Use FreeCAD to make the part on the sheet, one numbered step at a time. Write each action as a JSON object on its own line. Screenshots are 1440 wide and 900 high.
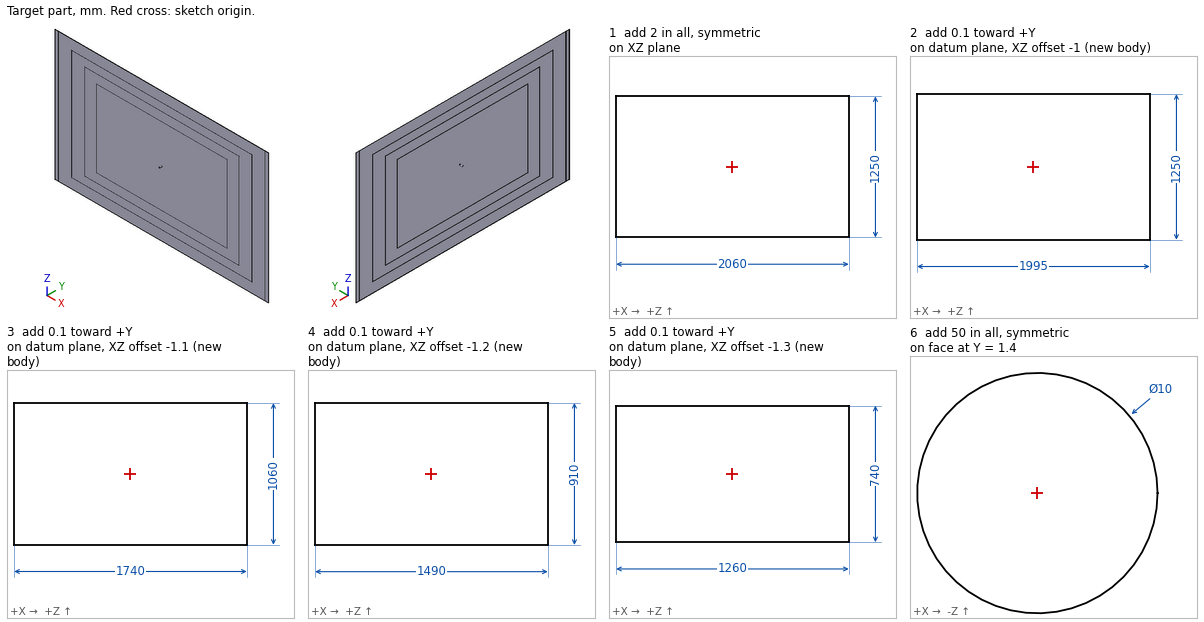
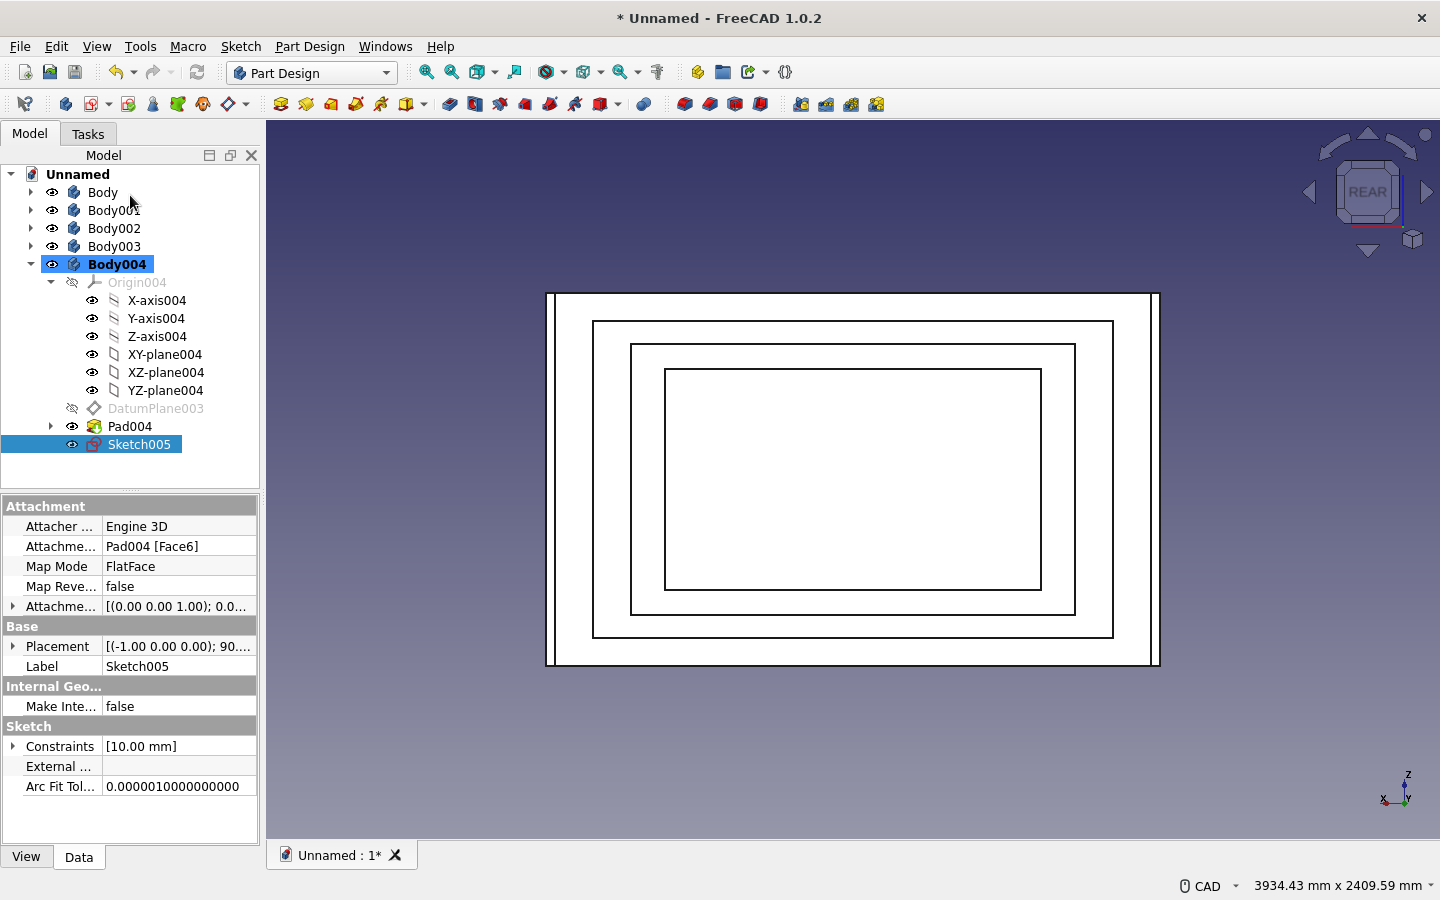
{"action": "left_click", "coordinate": [281, 104]}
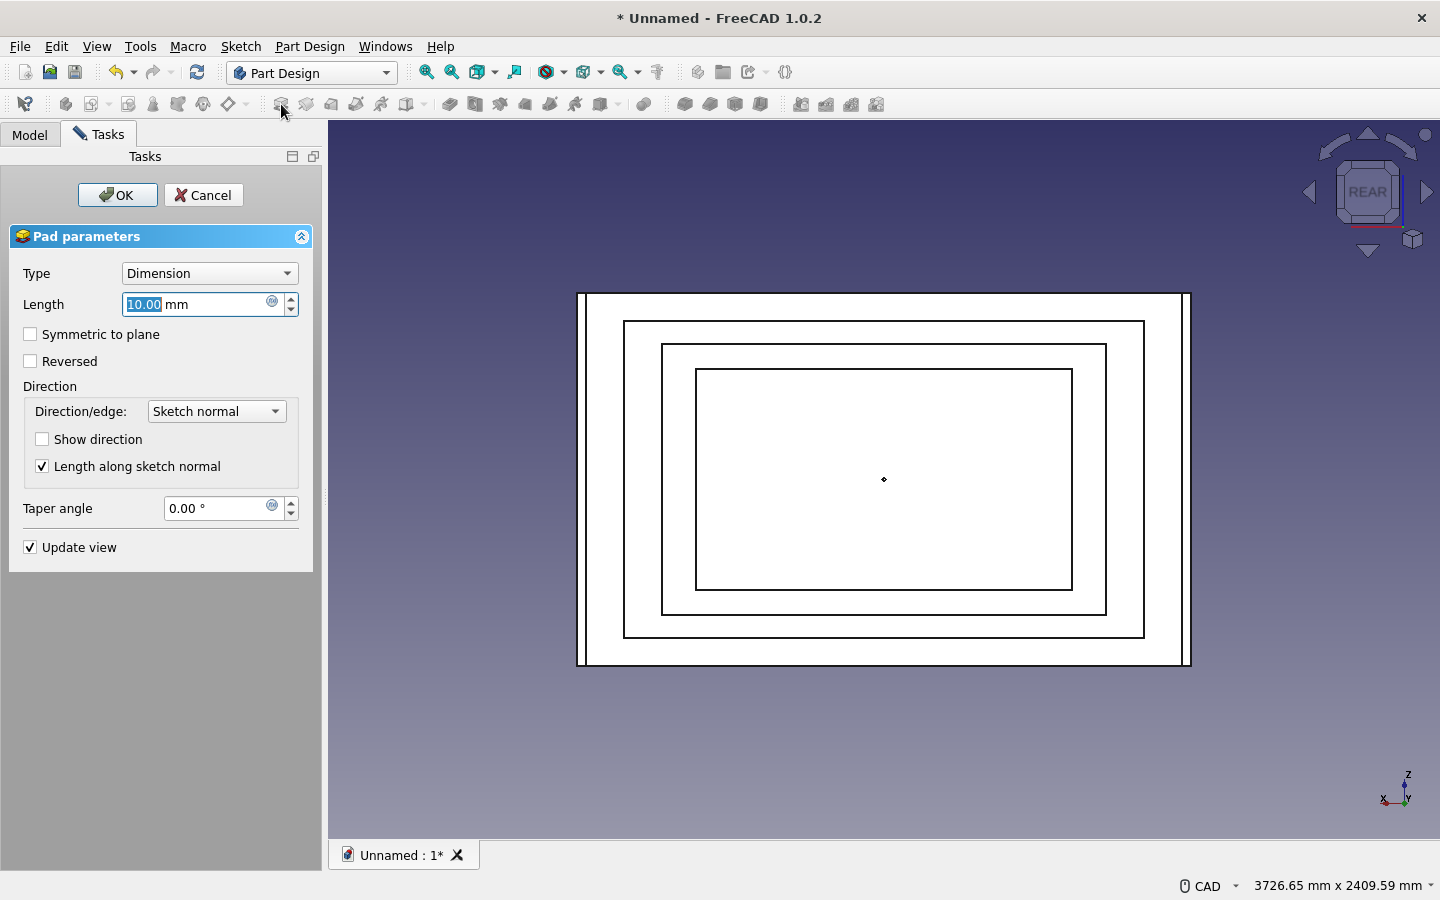
{"action": "type", "text": "50"}
{"action": "key", "text": "Tab"}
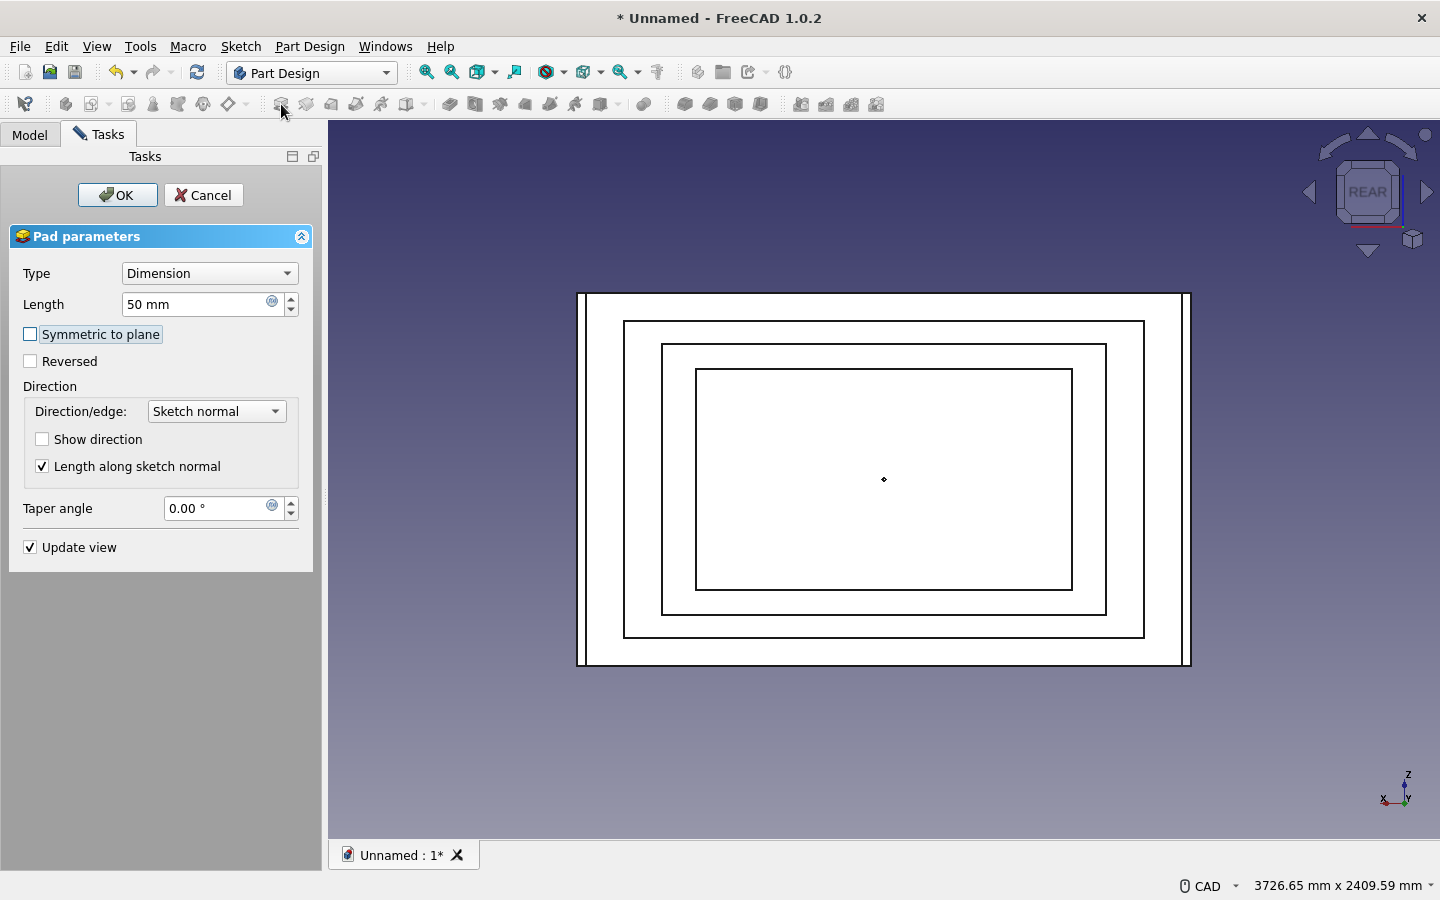
{"action": "left_click", "coordinate": [31, 334]}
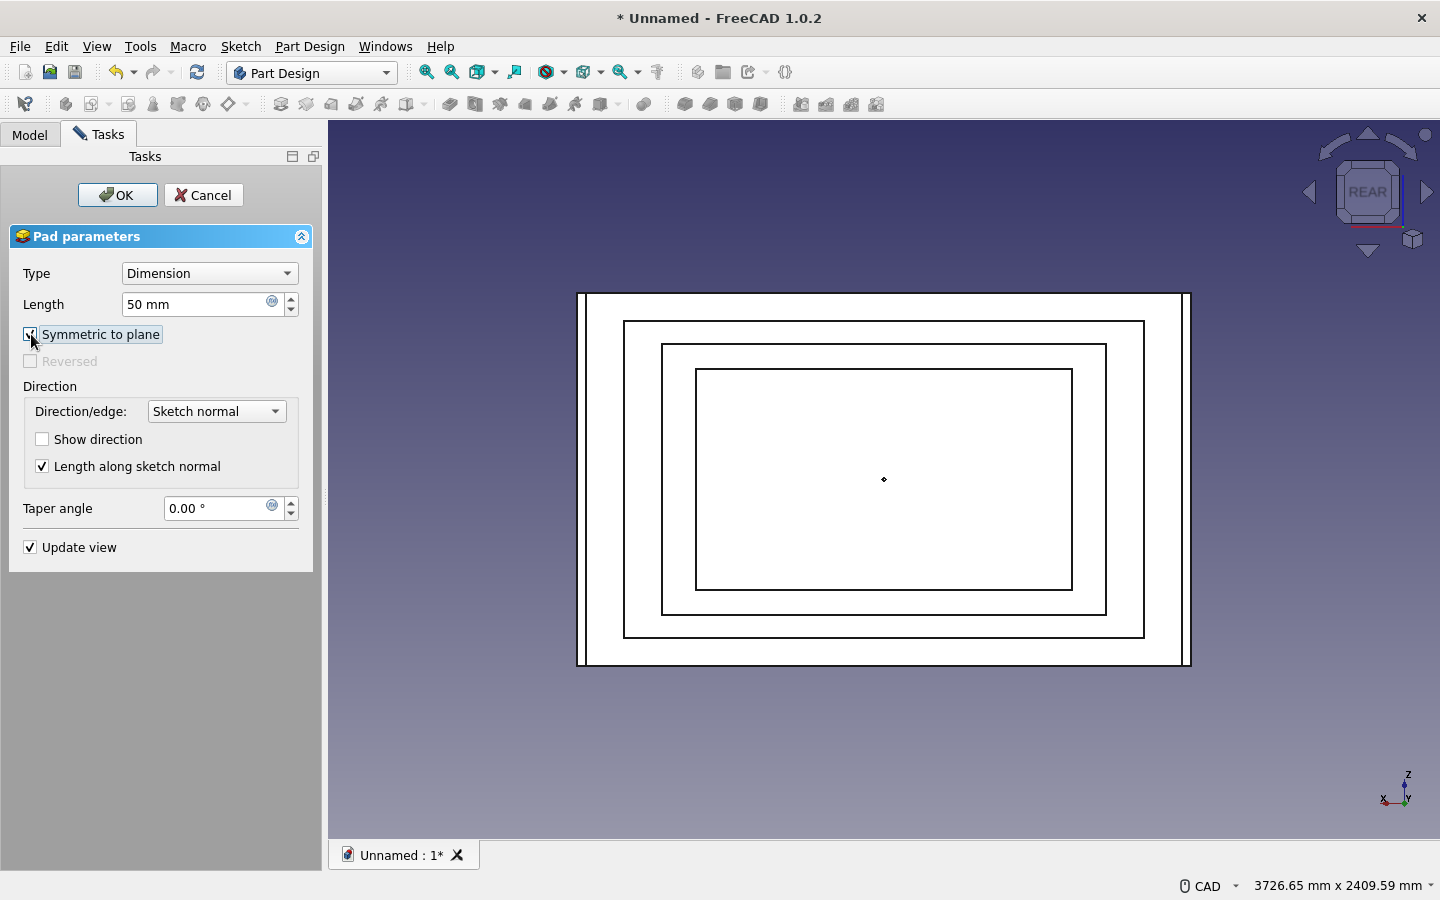
{"action": "left_click", "coordinate": [118, 195]}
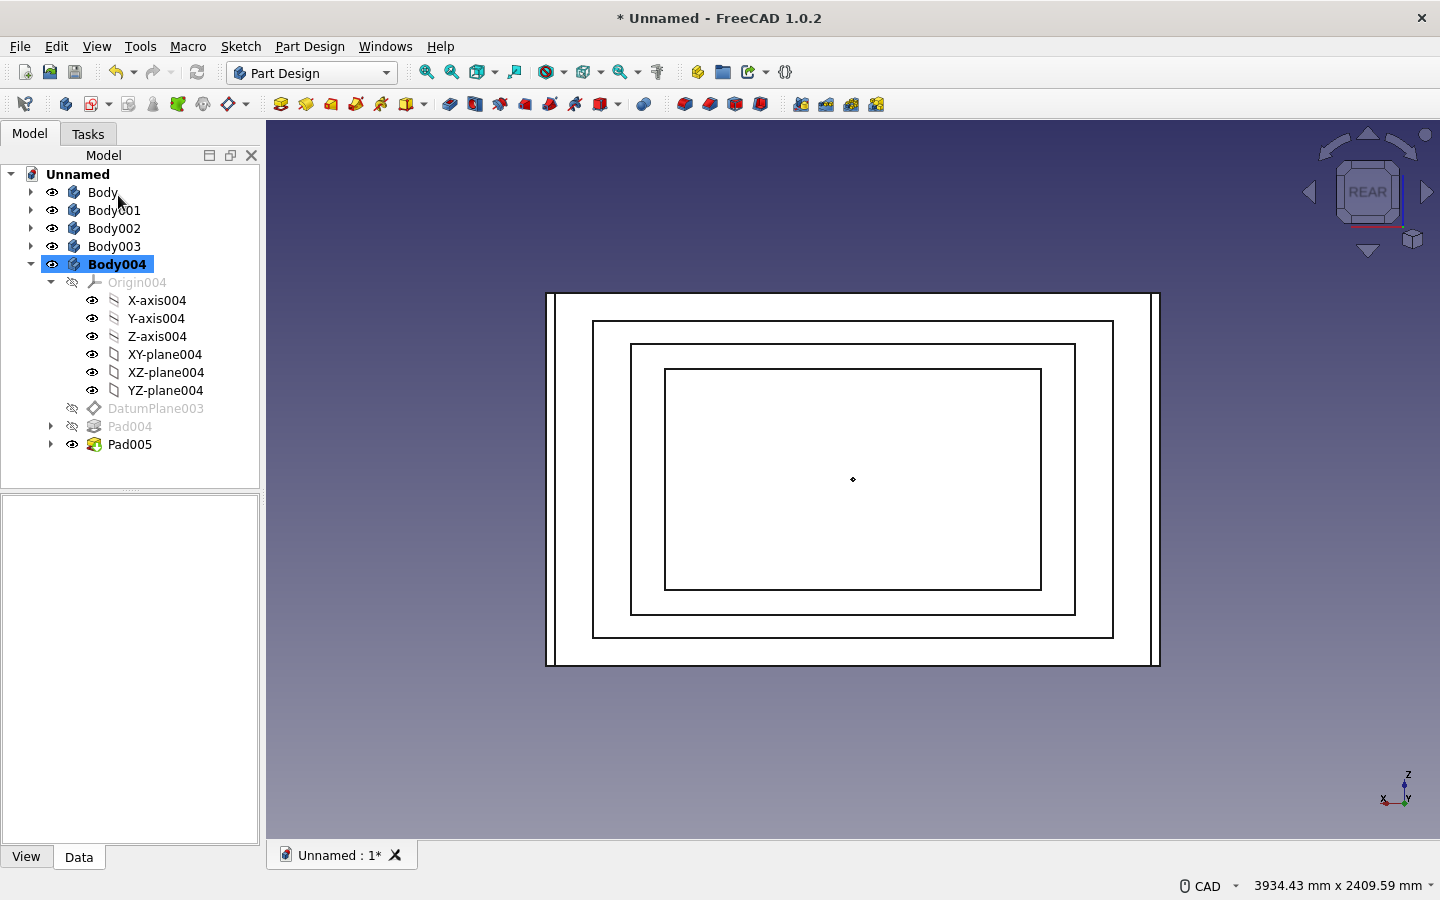
{"action": "key", "text": "0"}